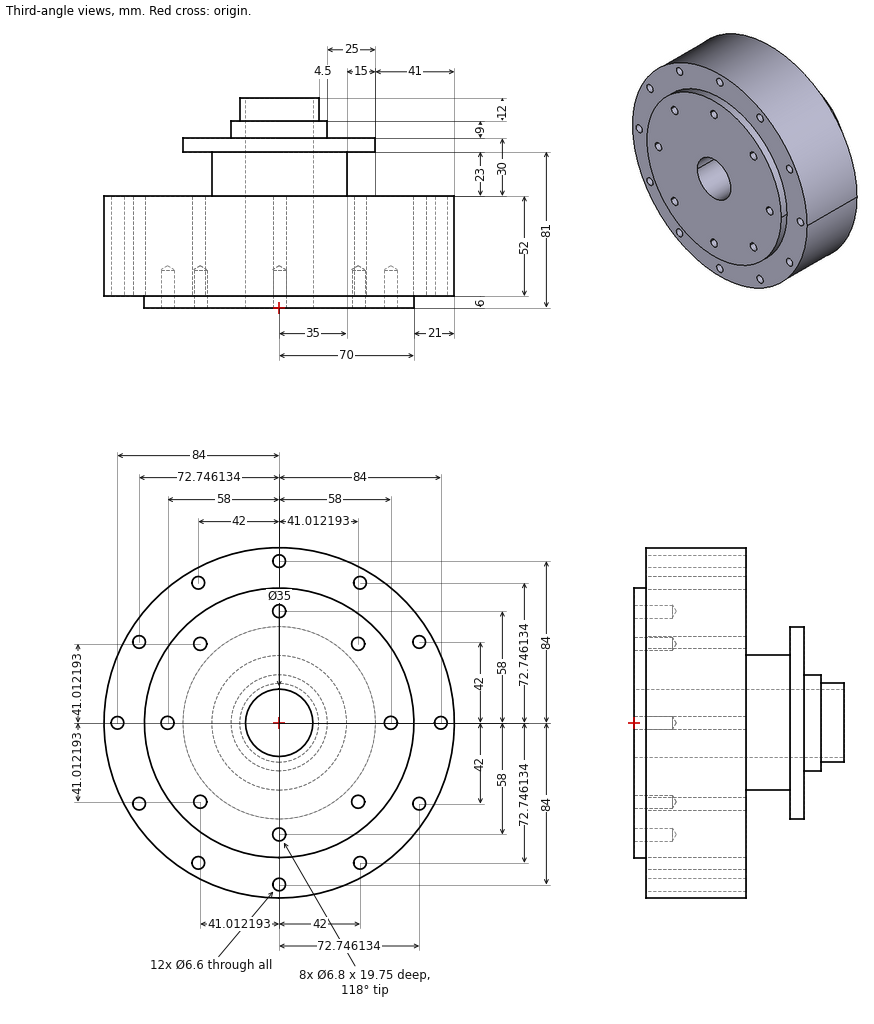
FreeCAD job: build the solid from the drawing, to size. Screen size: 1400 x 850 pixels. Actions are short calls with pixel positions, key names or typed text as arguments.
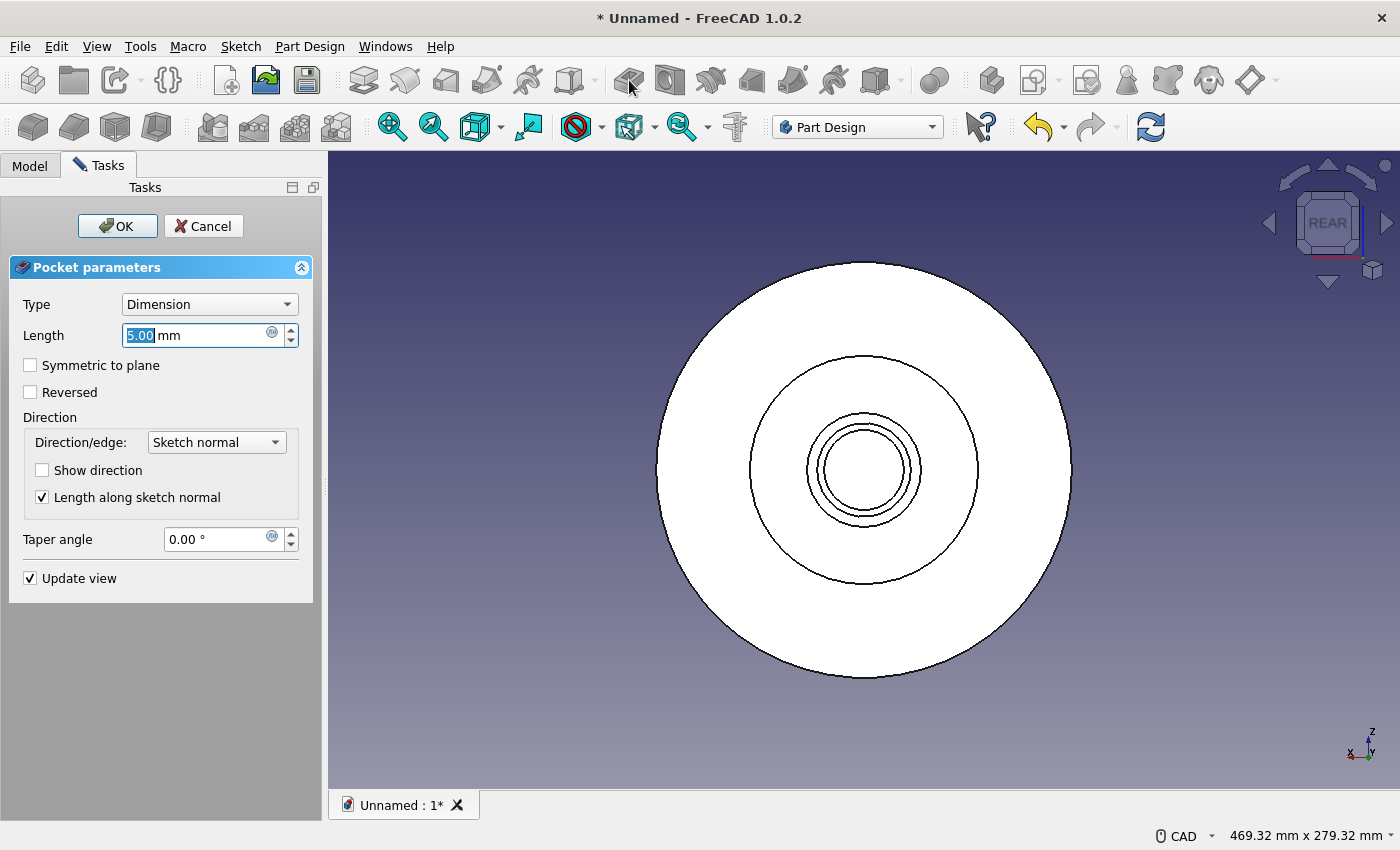
click(210, 304)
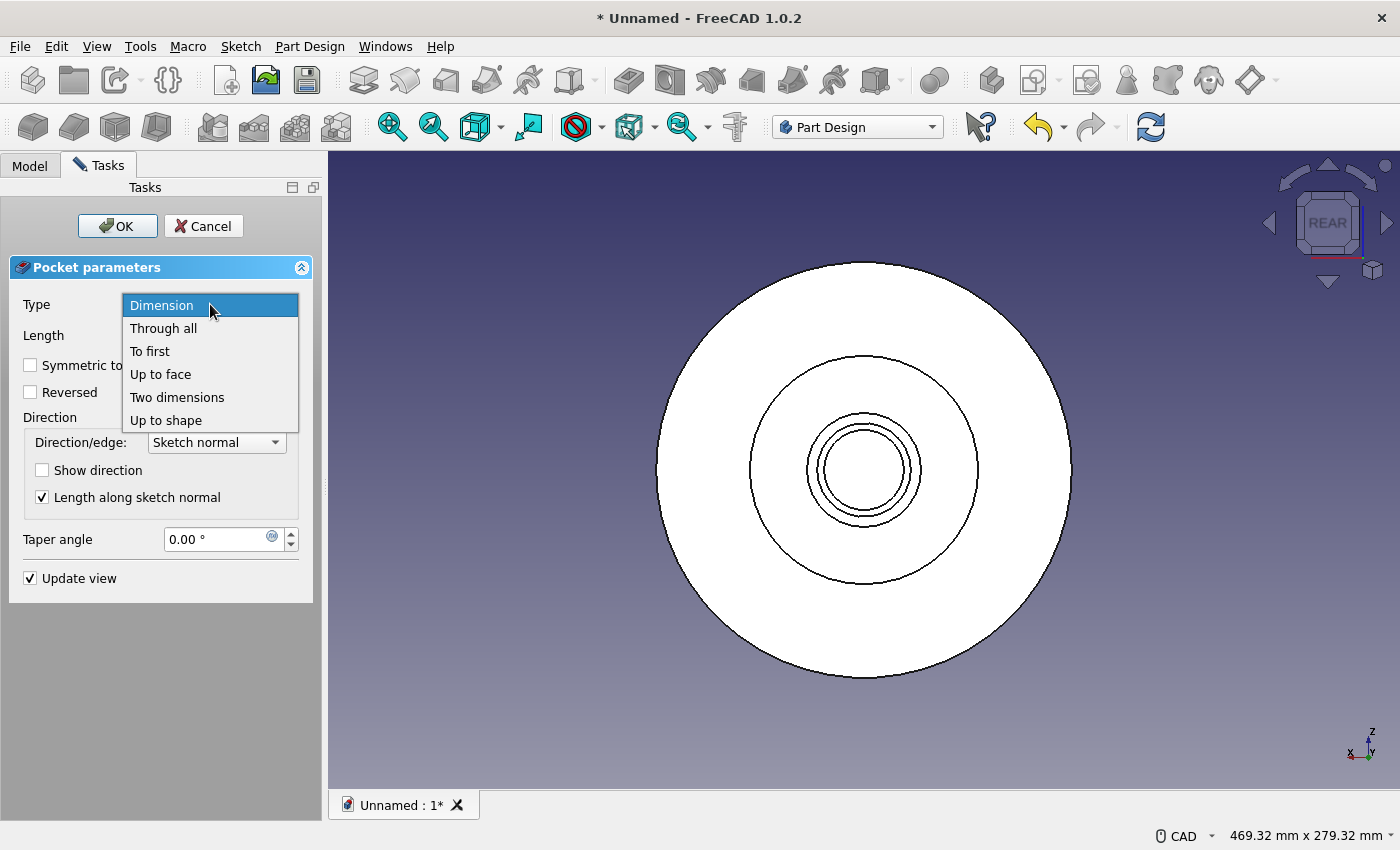
click(208, 328)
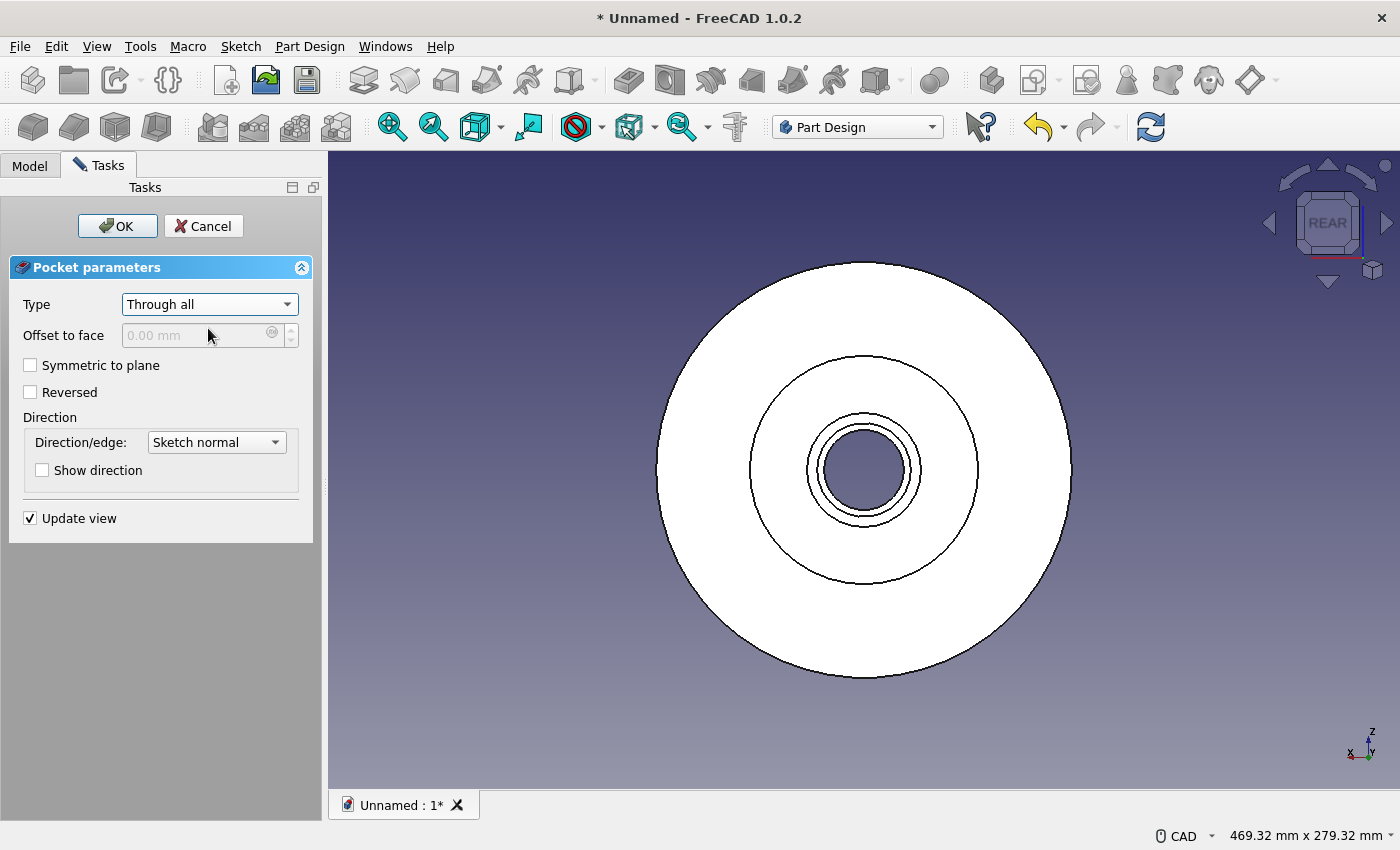
click(118, 226)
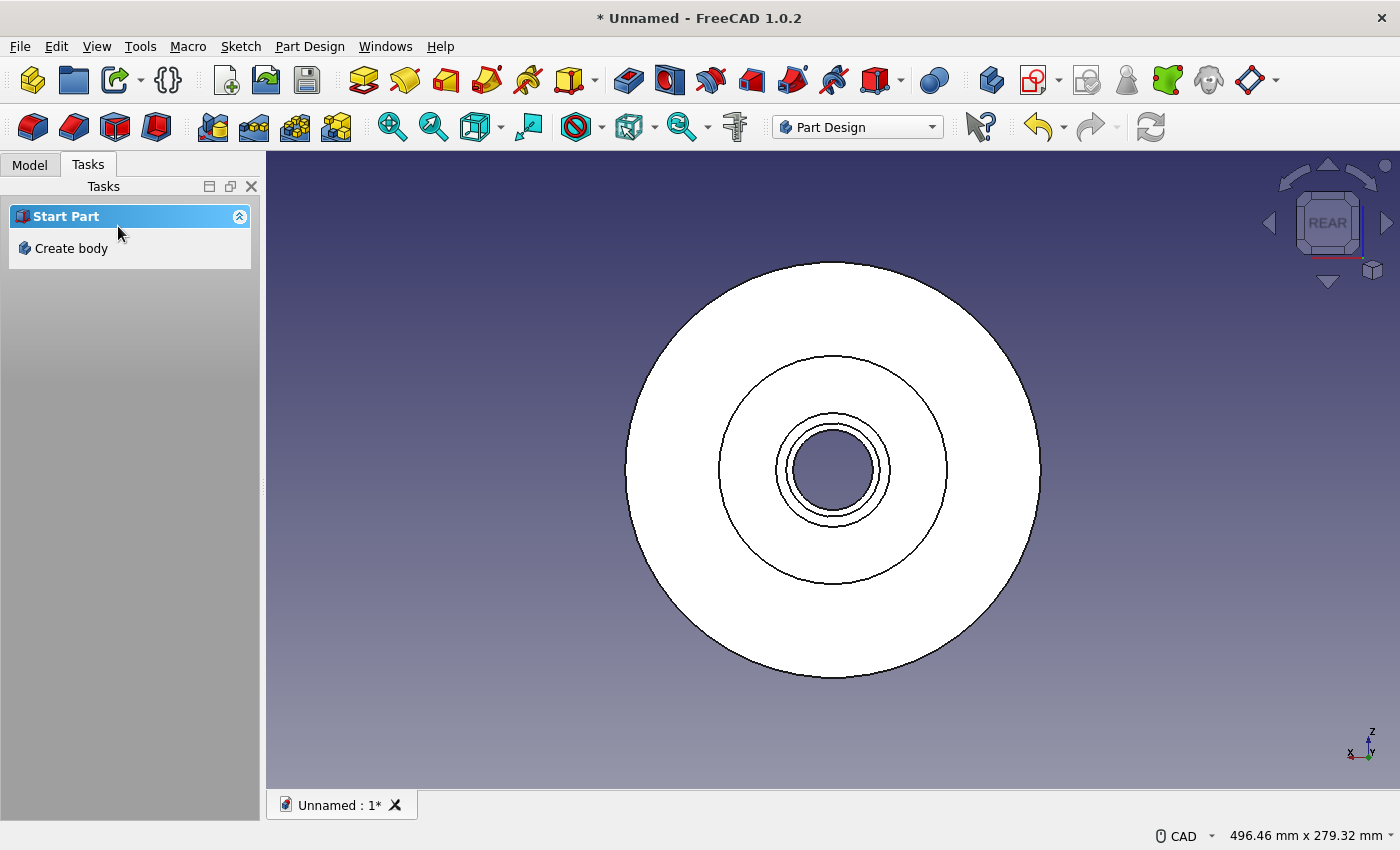
click(714, 350)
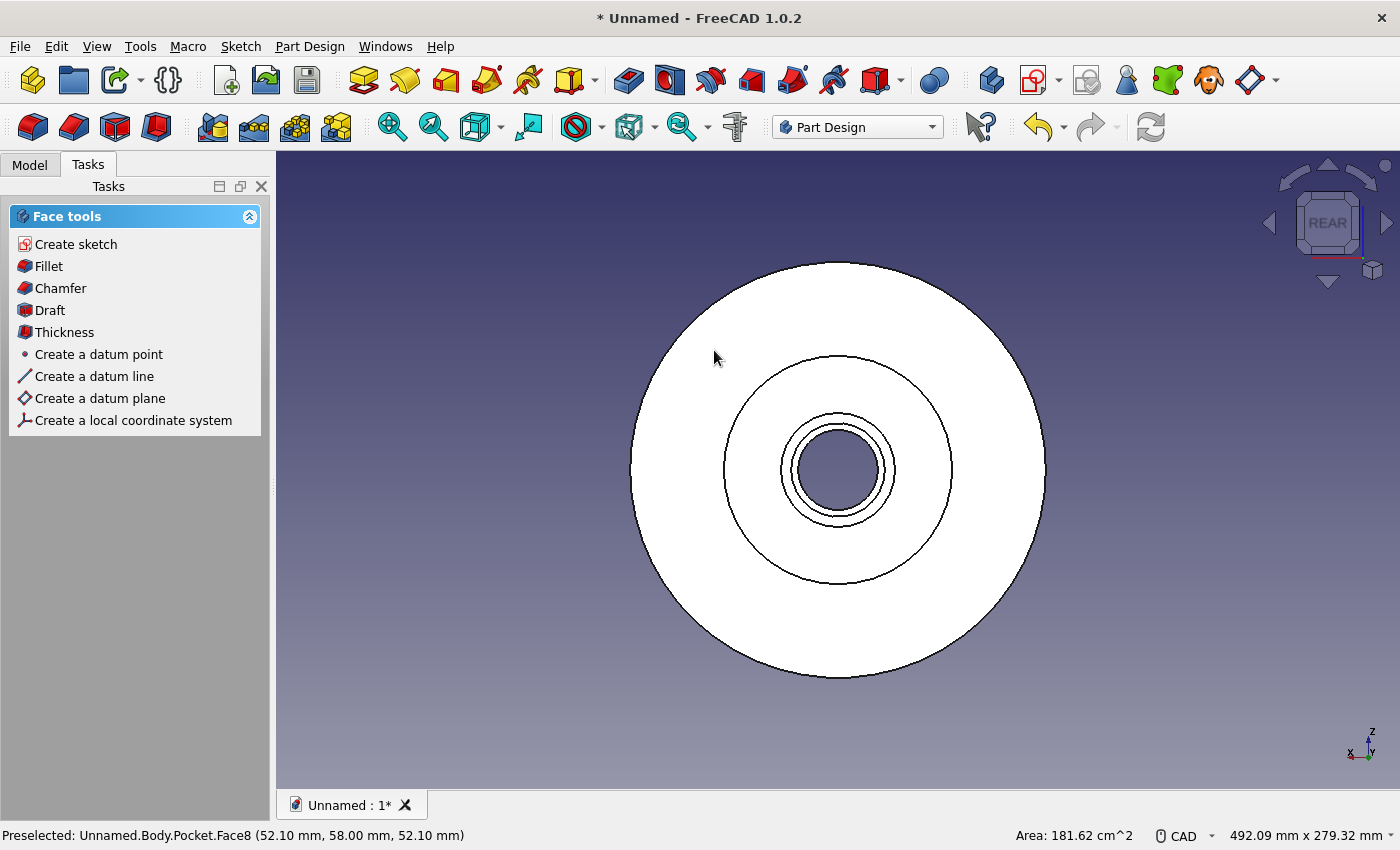
click(1032, 80)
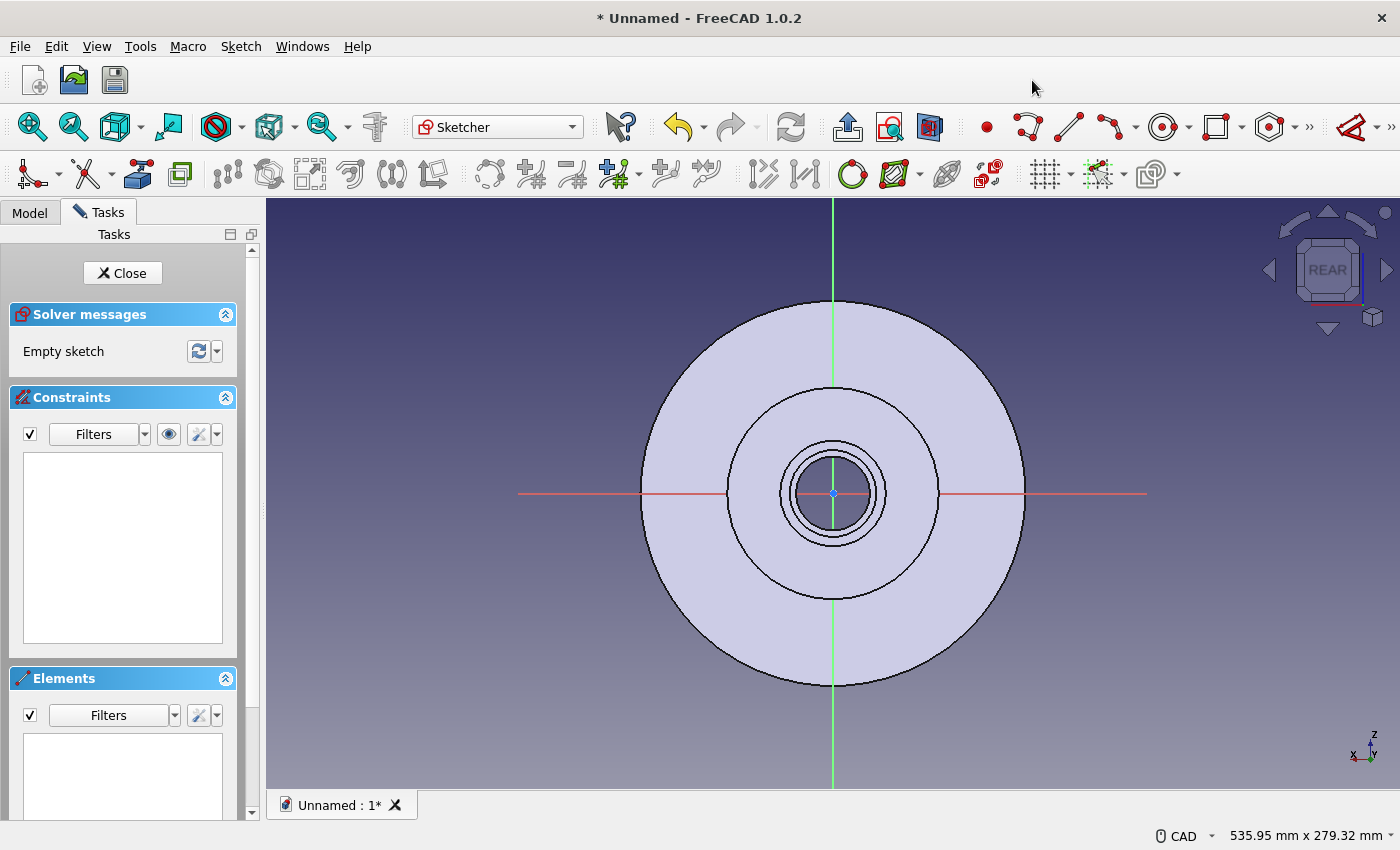
key(q)
key(s)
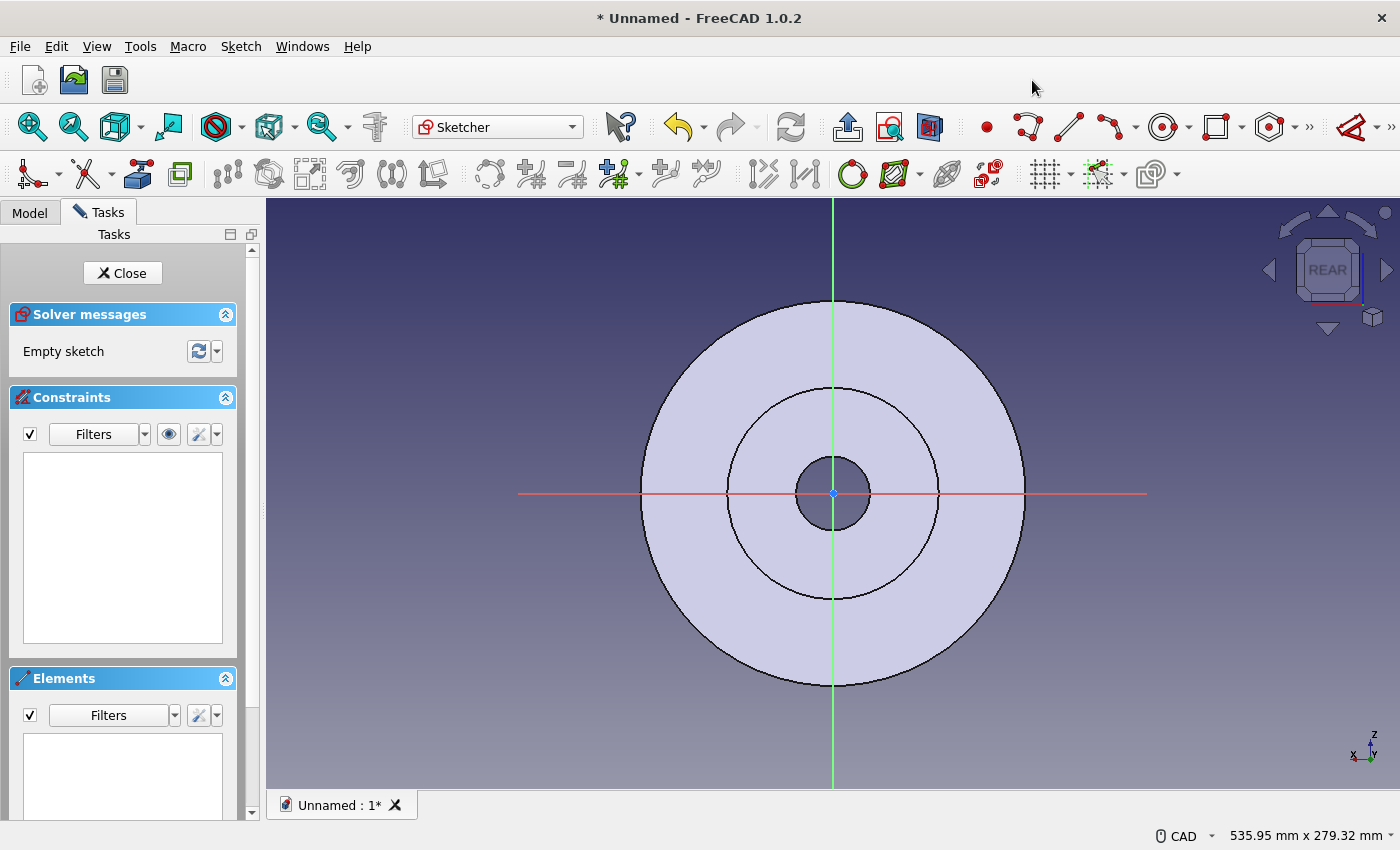
key(g)
key(c)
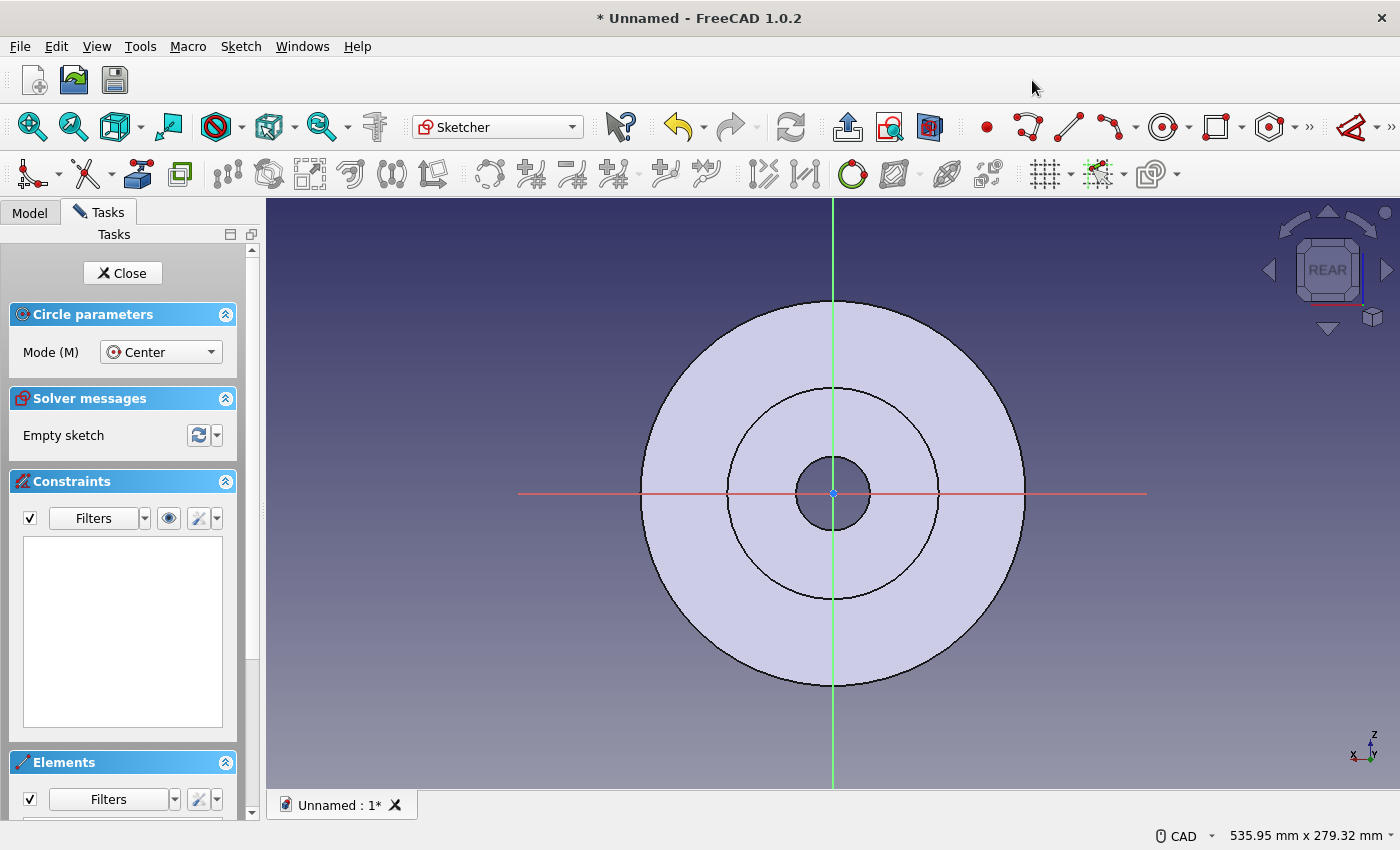
scroll(833, 671, up, 6)